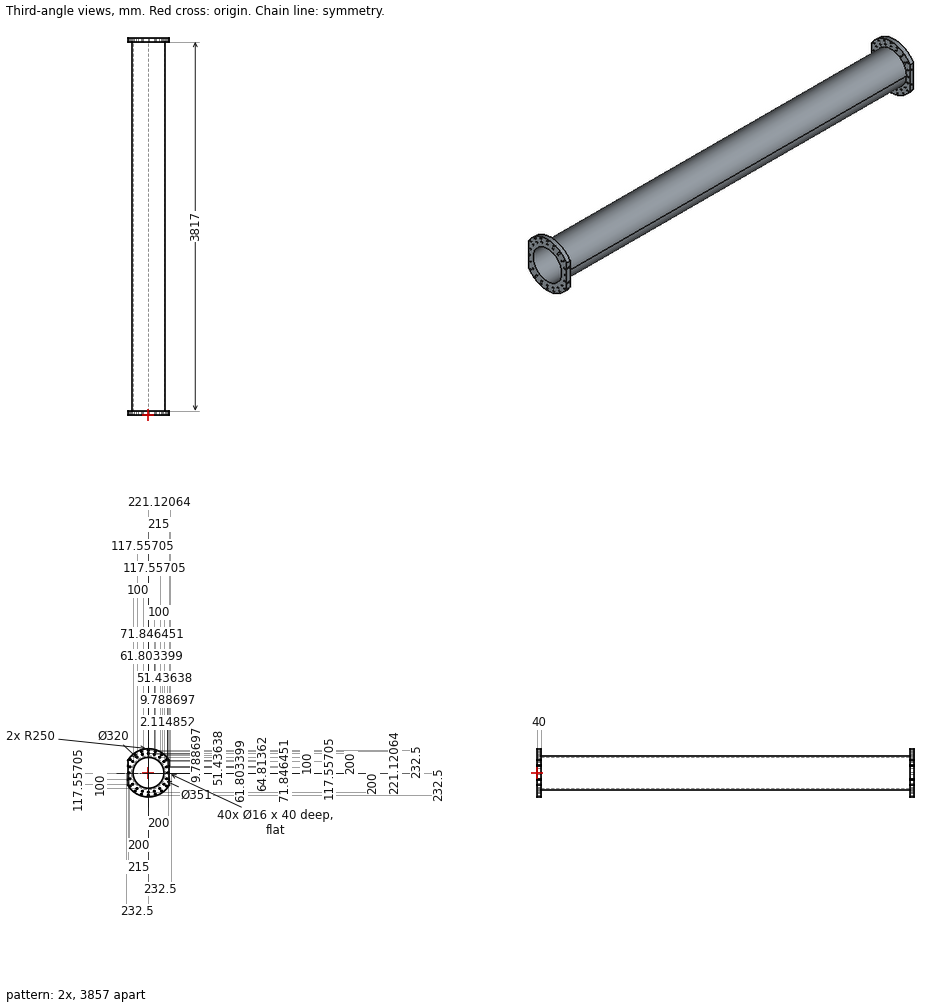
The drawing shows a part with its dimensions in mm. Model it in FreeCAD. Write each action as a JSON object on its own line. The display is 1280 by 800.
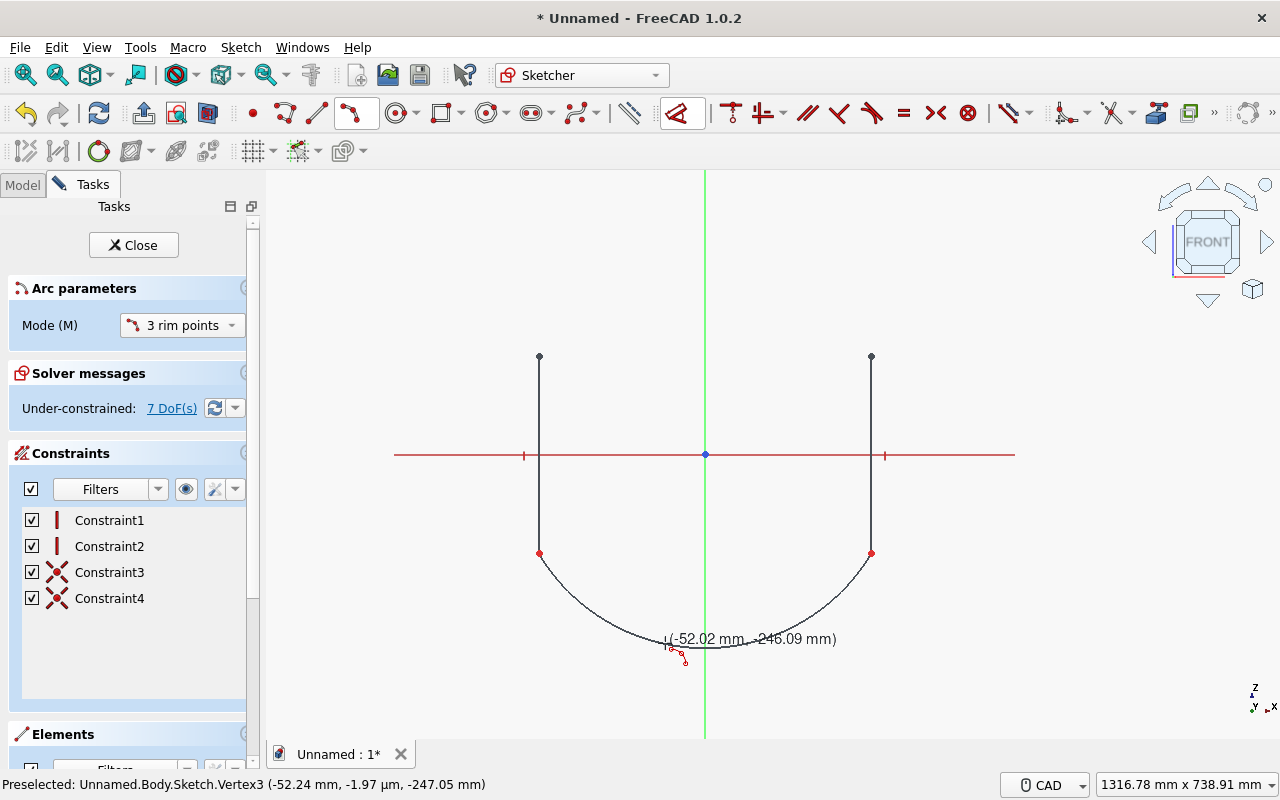
{"action": "left_click", "coordinate": [539, 357]}
{"action": "left_click", "coordinate": [871, 357]}
{"action": "left_click", "coordinate": [745, 266]}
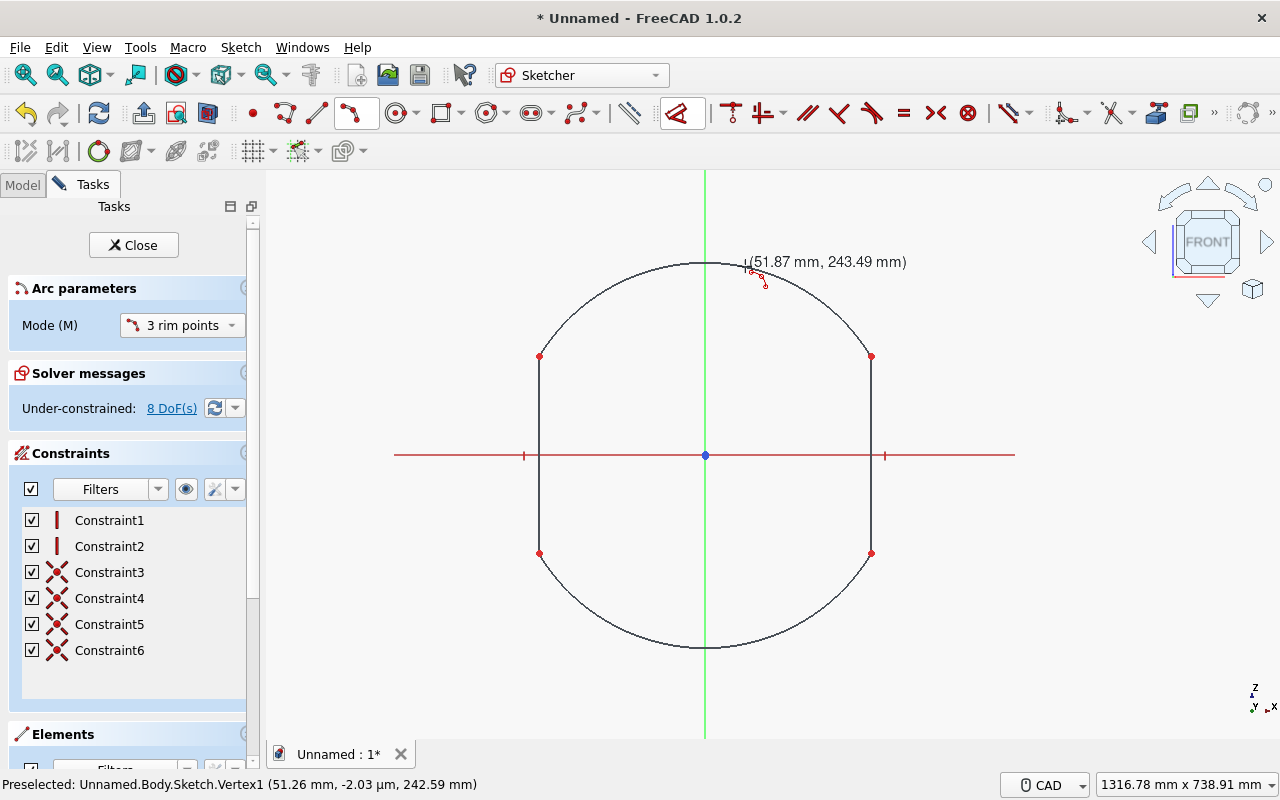
{"action": "left_click", "coordinate": [396, 114]}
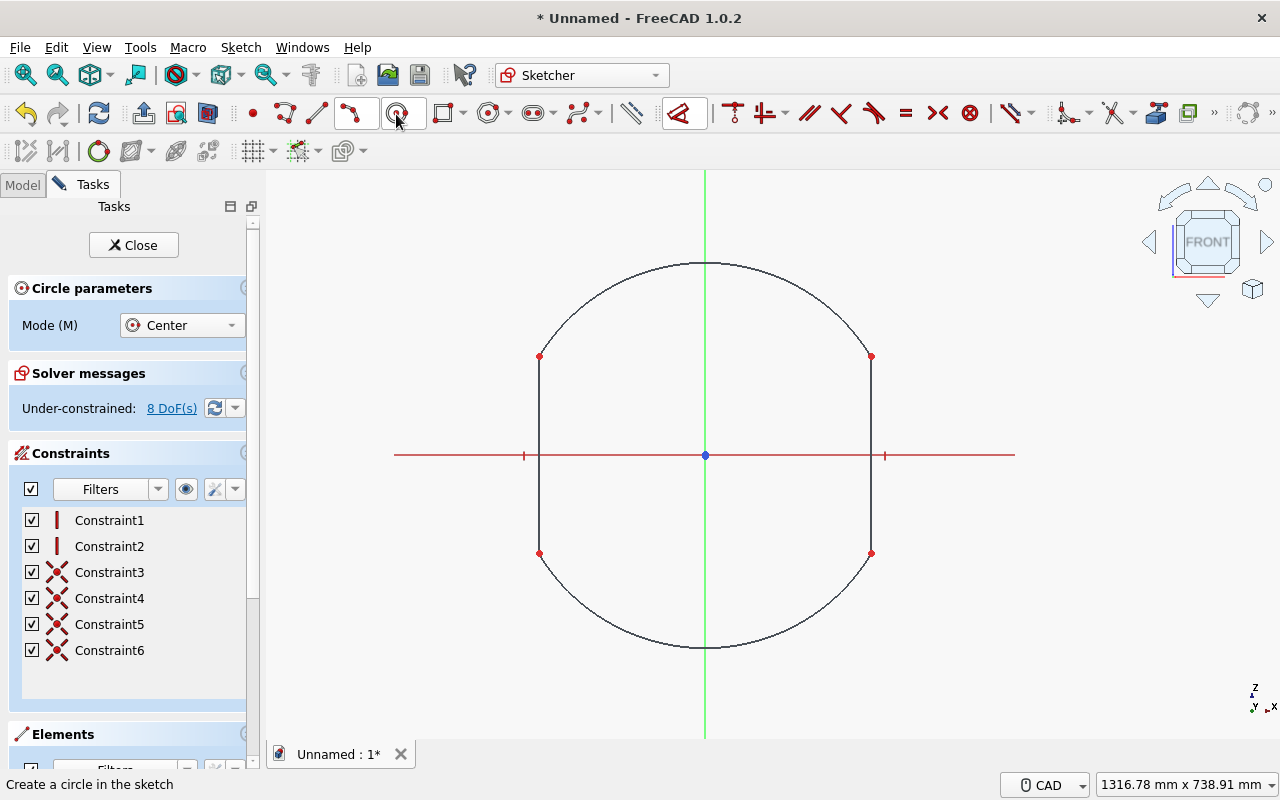
{"action": "left_click", "coordinate": [705, 454]}
{"action": "mouse_move", "coordinate": [792, 367]}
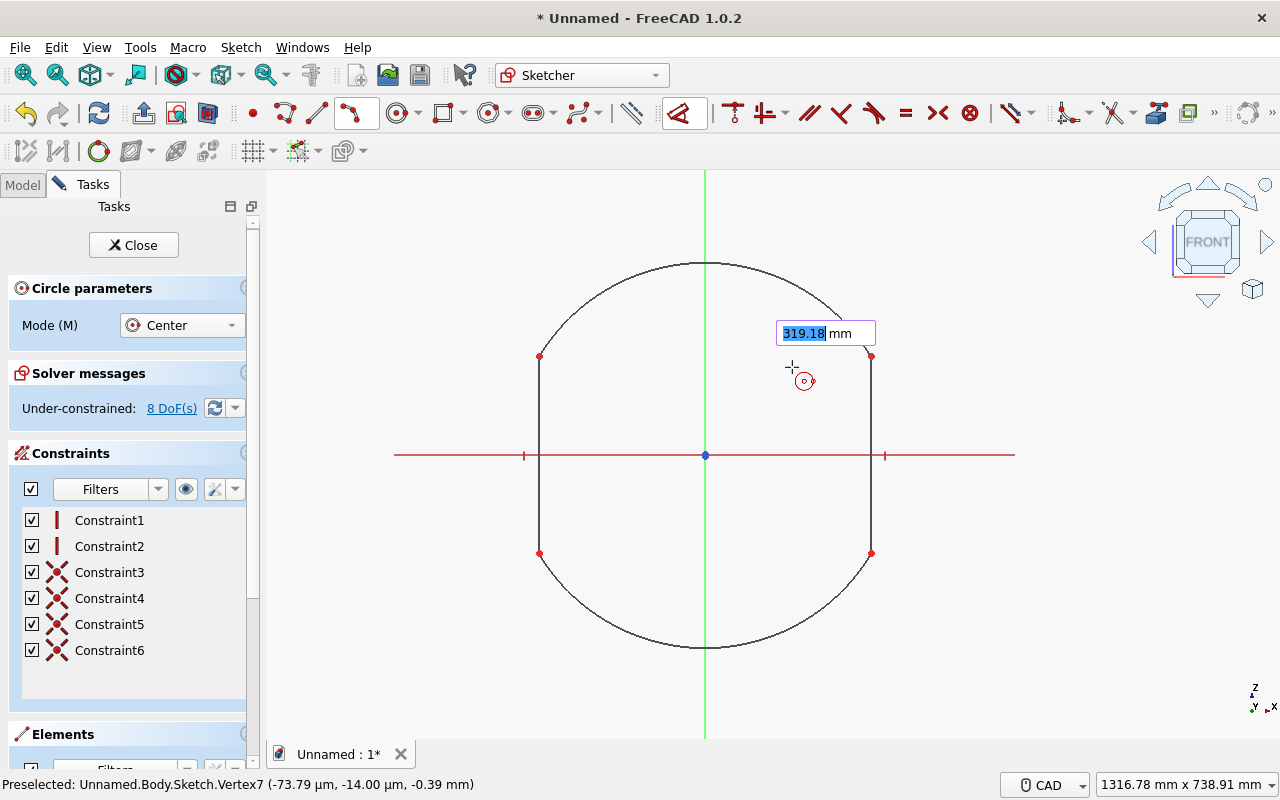
{"action": "type", "text": "320"}
{"action": "key", "text": "Return"}
{"action": "key", "text": "Escape"}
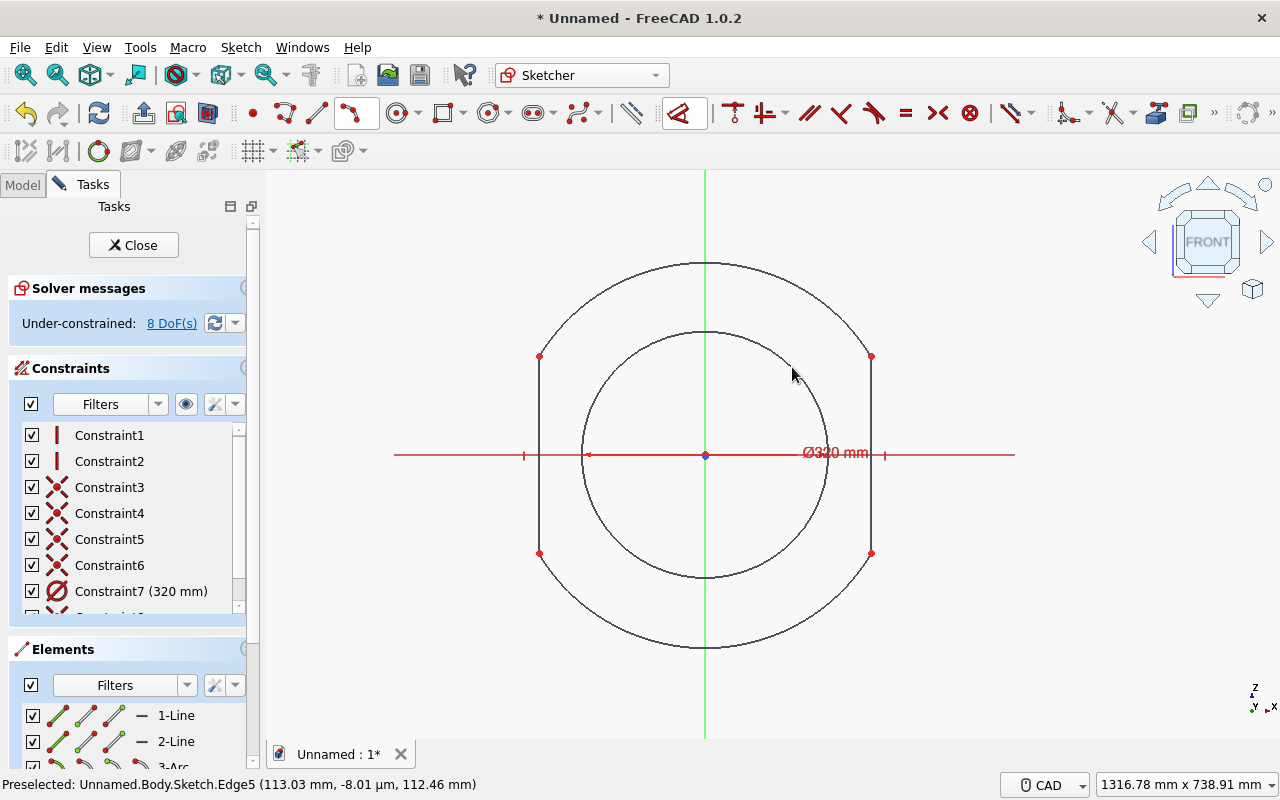
{"action": "left_click", "coordinate": [792, 367]}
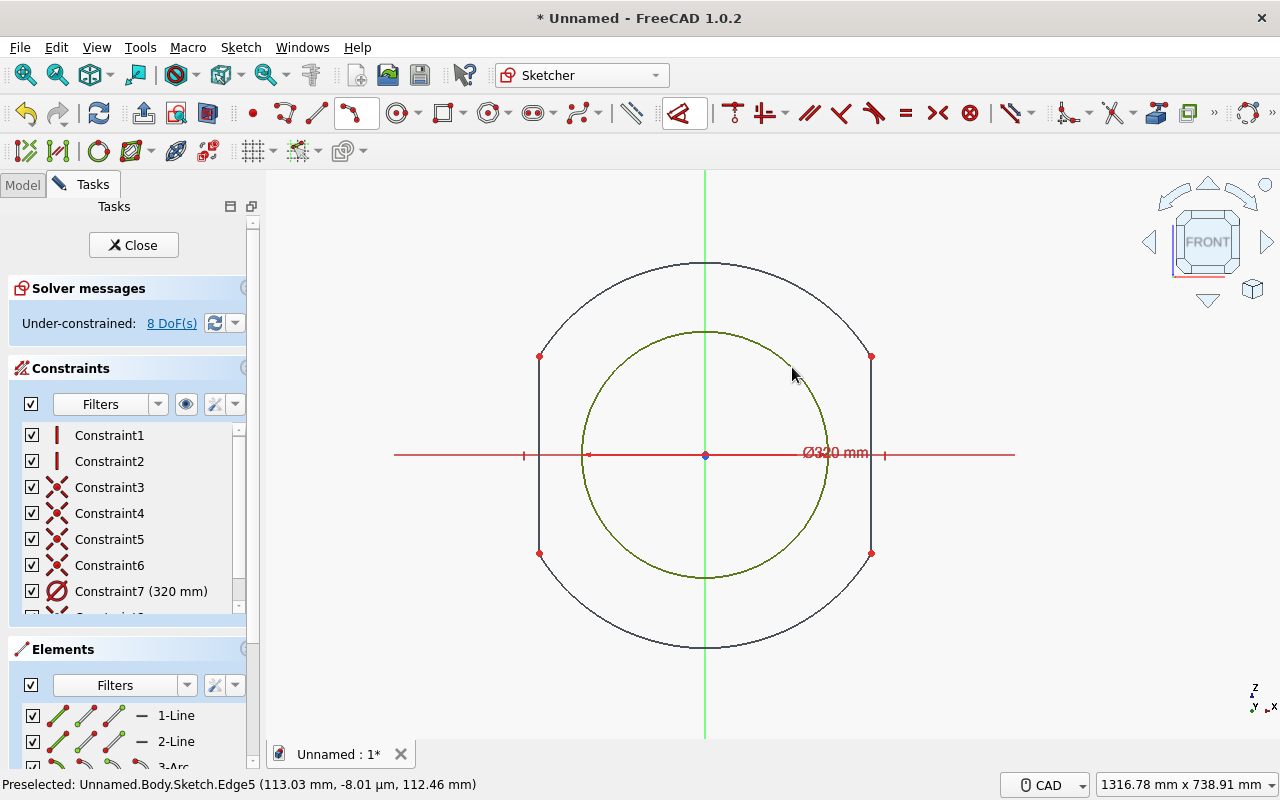
{"action": "left_click", "coordinate": [783, 279]}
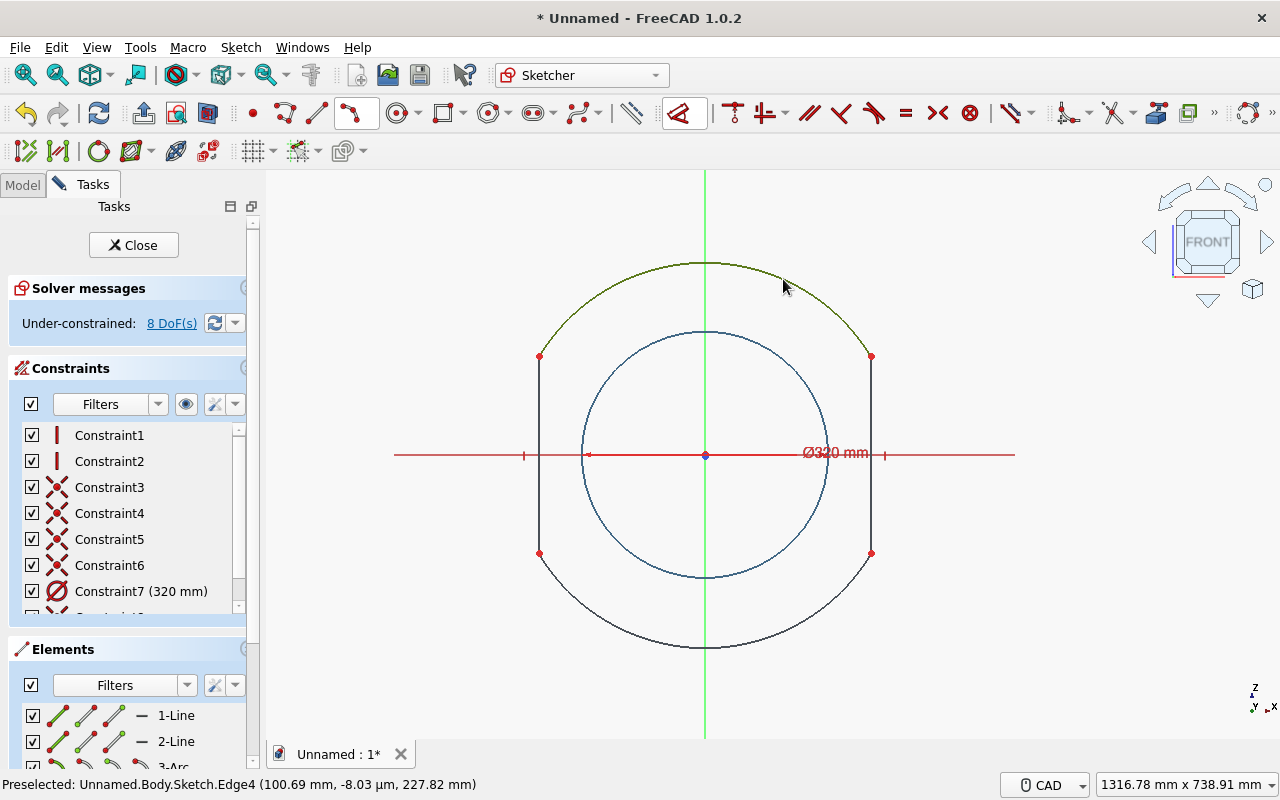
{"action": "left_click", "coordinate": [734, 114]}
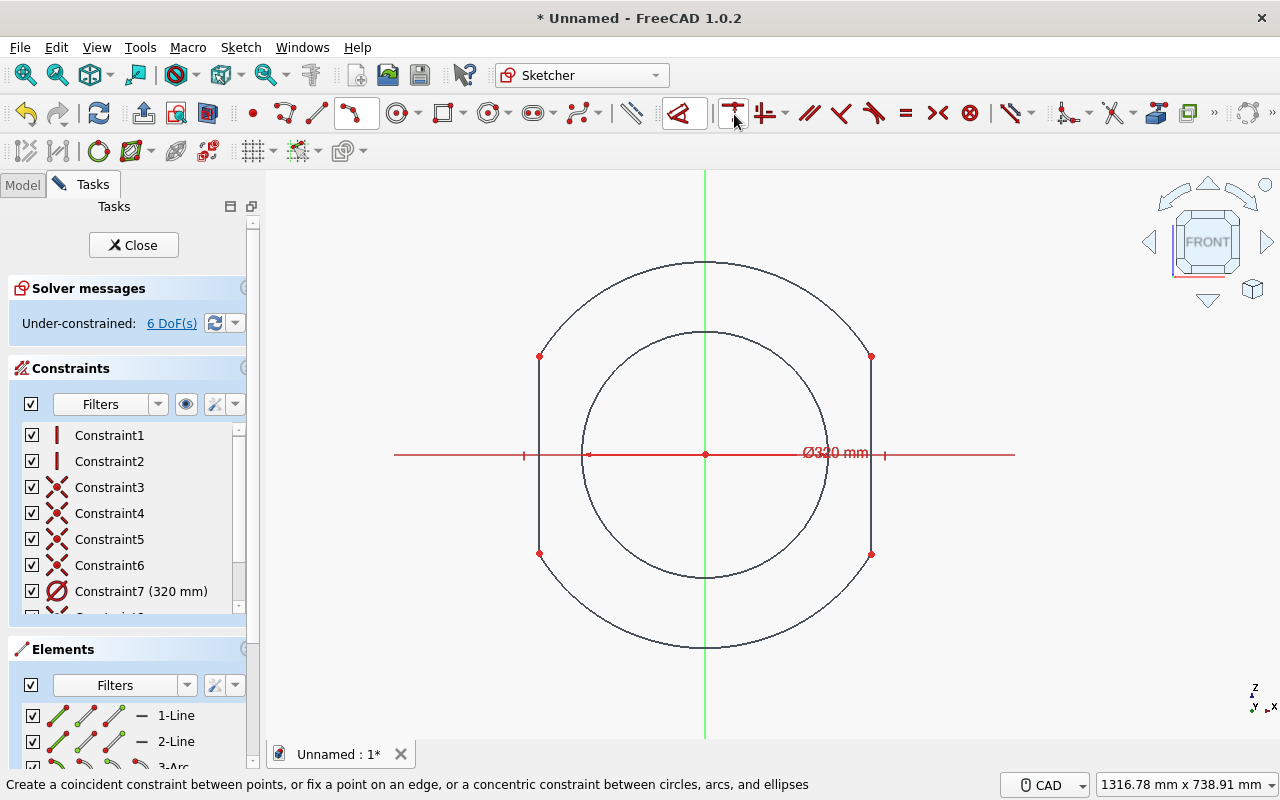
{"action": "left_click_drag", "start_coordinate": [695, 444], "coordinate": [715, 465]}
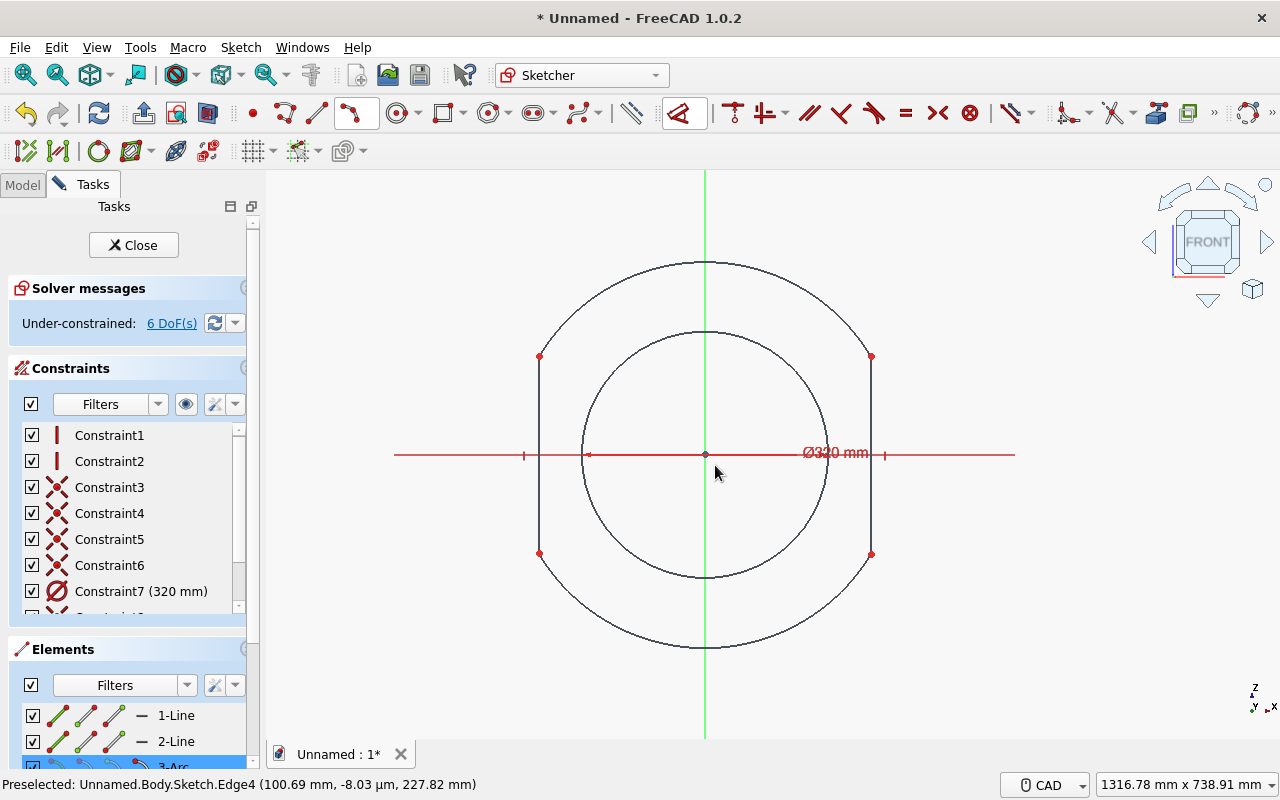
{"action": "left_click", "coordinate": [734, 114]}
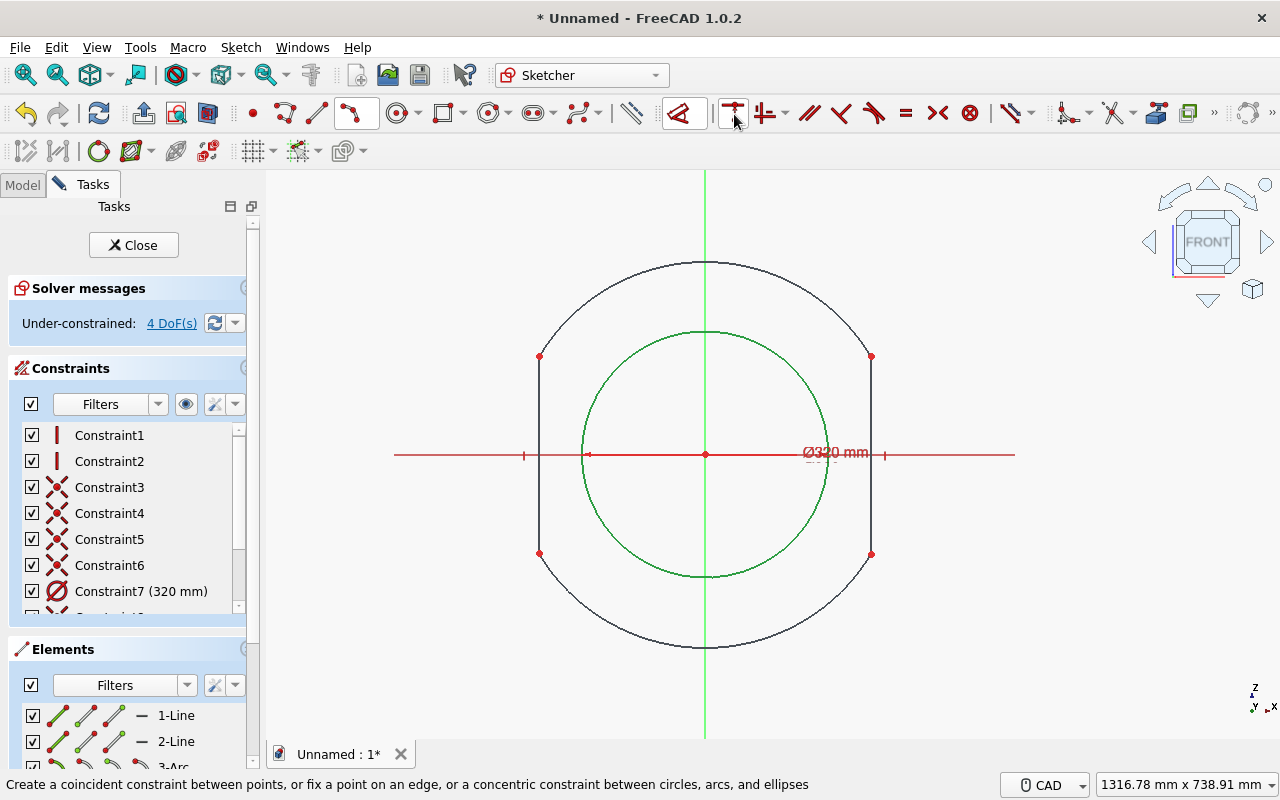
{"action": "left_click", "coordinate": [628, 632]}